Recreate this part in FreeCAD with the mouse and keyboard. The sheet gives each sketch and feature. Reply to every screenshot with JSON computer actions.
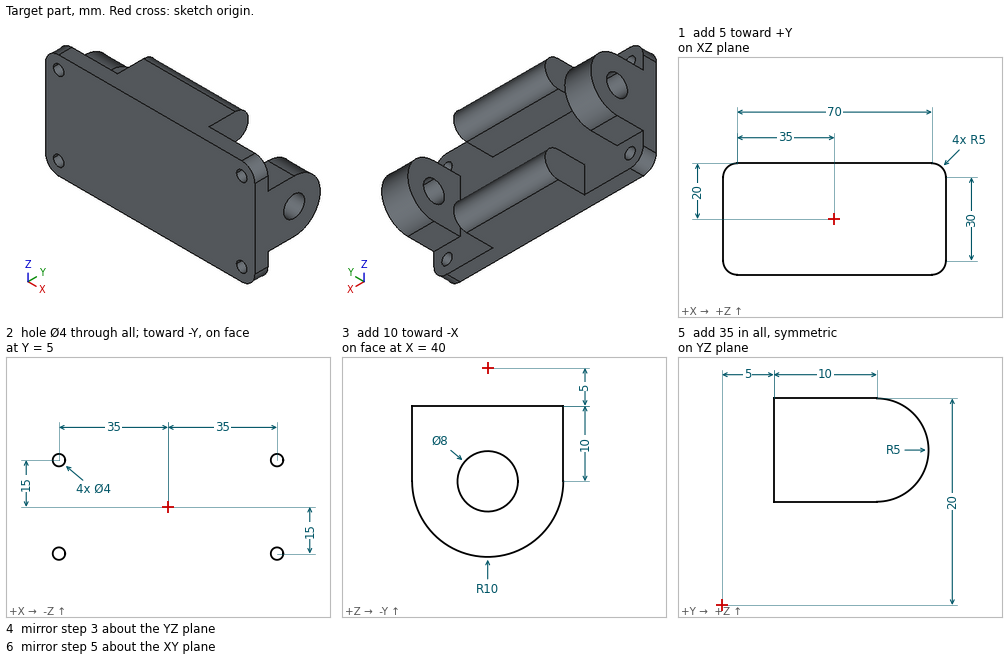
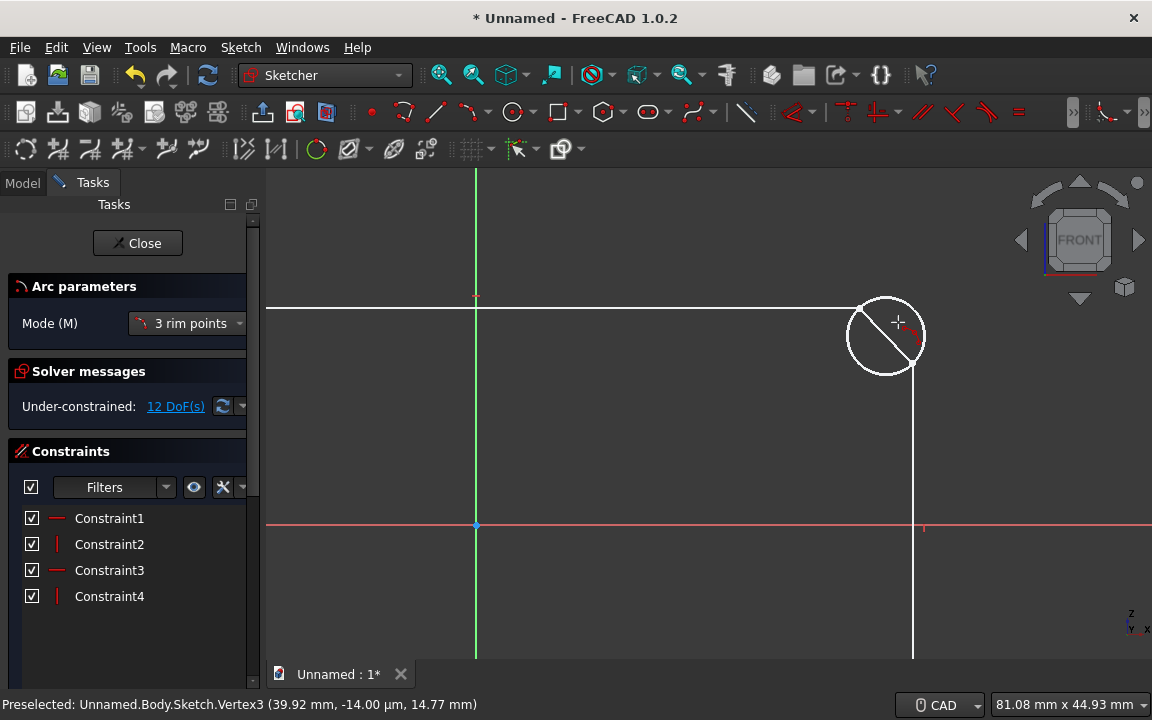
{"action": "left_click", "coordinate": [898, 323]}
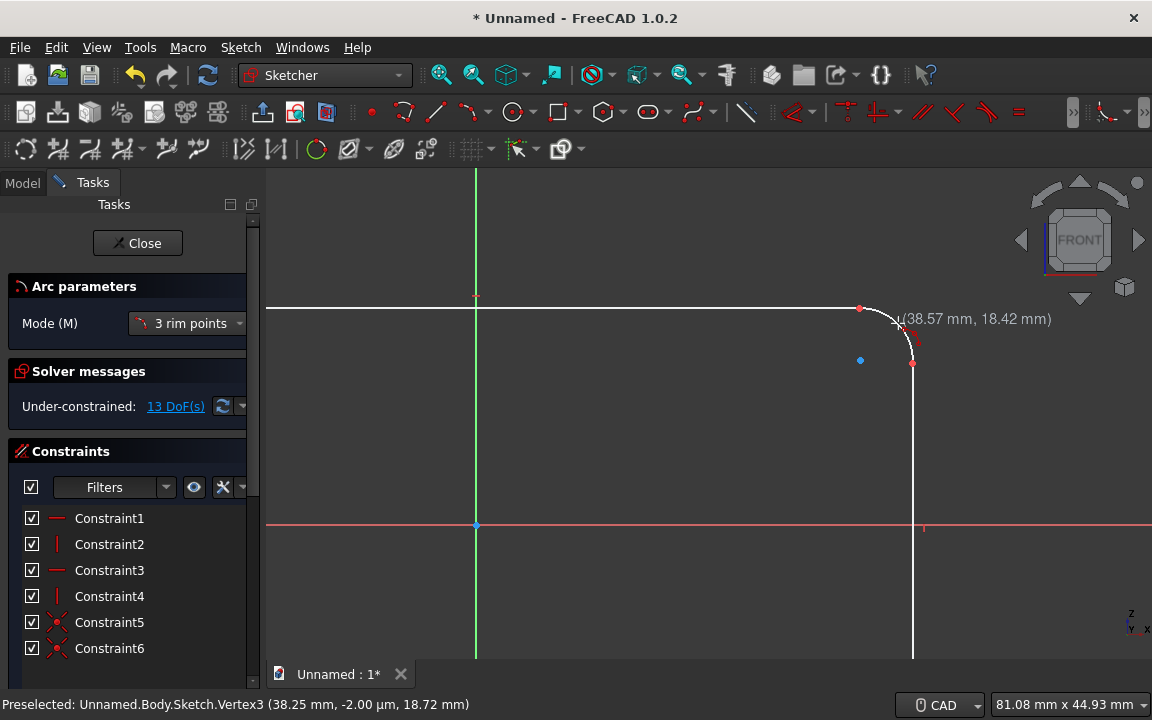
{"action": "scroll", "coordinate": [840, 278], "scroll_direction": "down", "scroll_amount": 3}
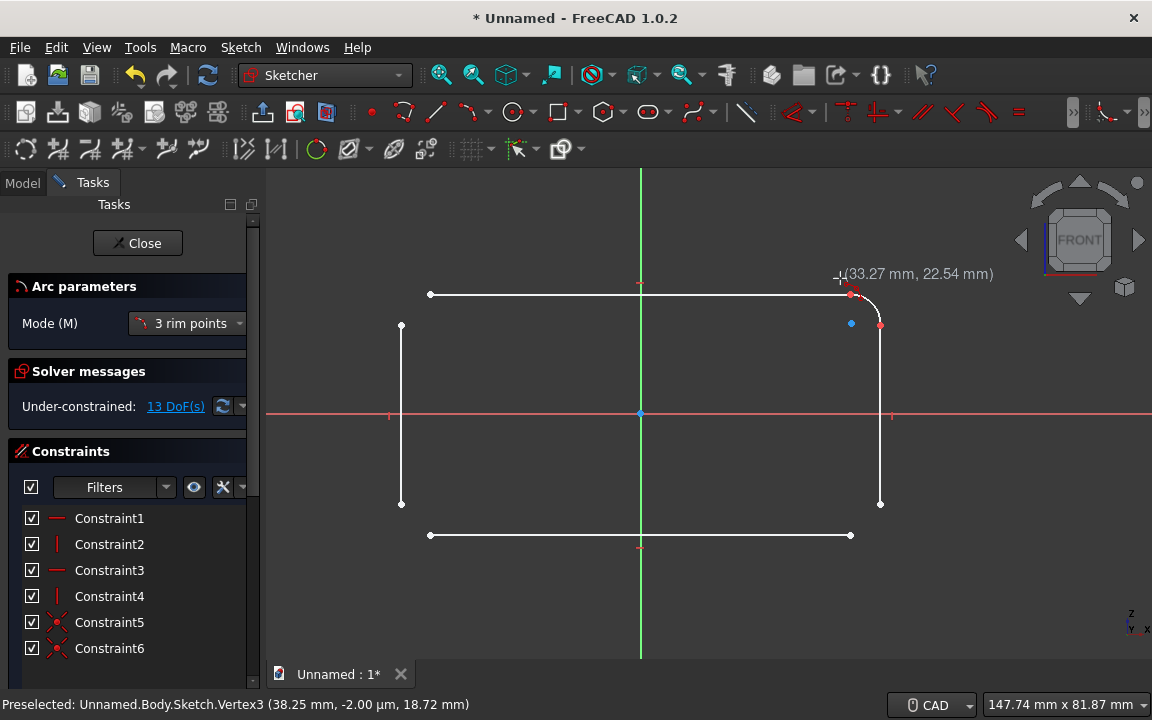
{"action": "left_click", "coordinate": [880, 505]}
{"action": "left_click", "coordinate": [851, 535]}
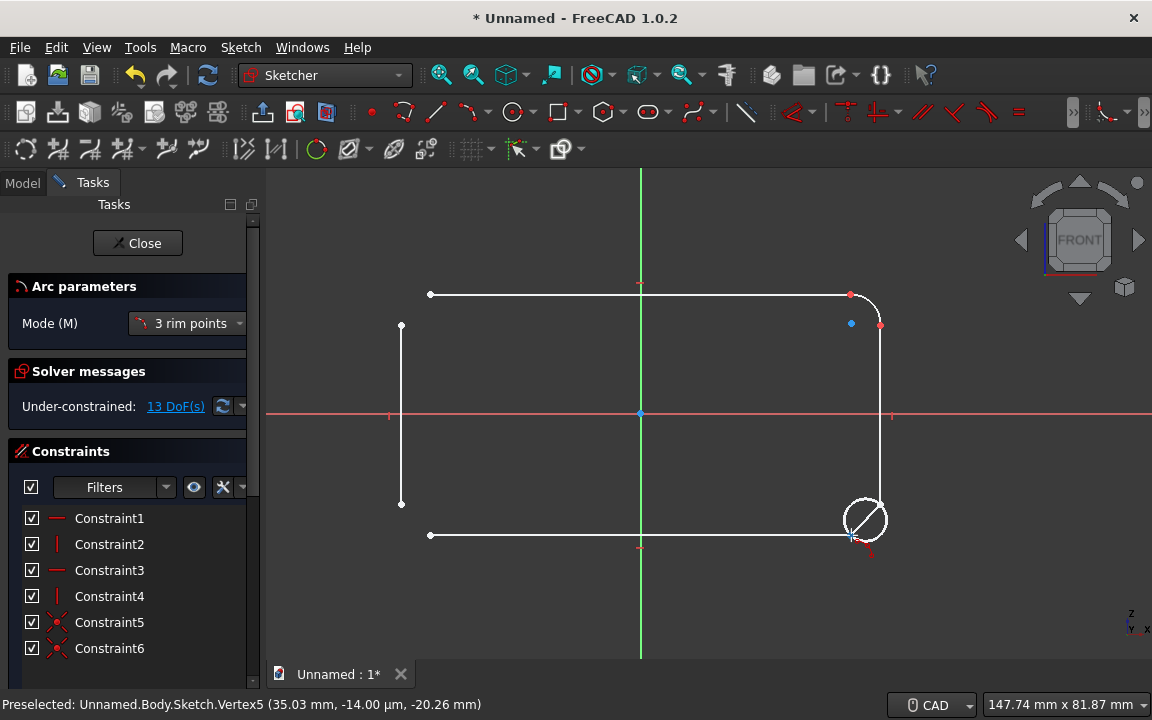
{"action": "scroll", "coordinate": [872, 525], "scroll_direction": "up", "scroll_amount": 3}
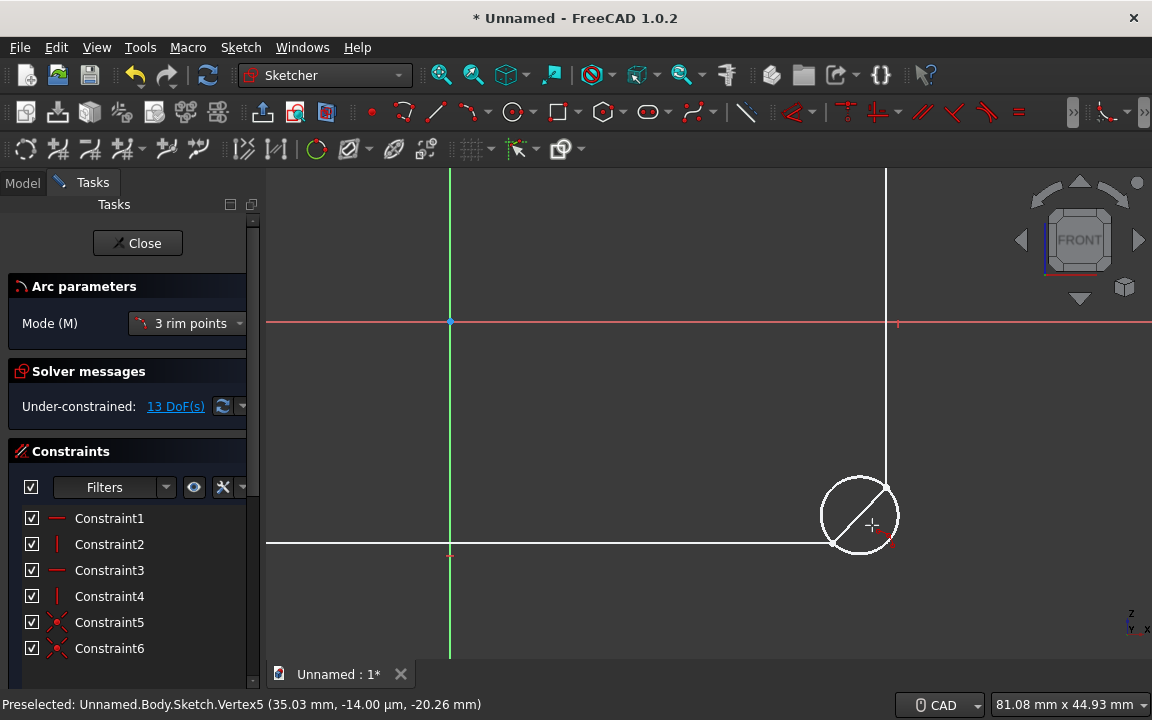
{"action": "left_click", "coordinate": [871, 524]}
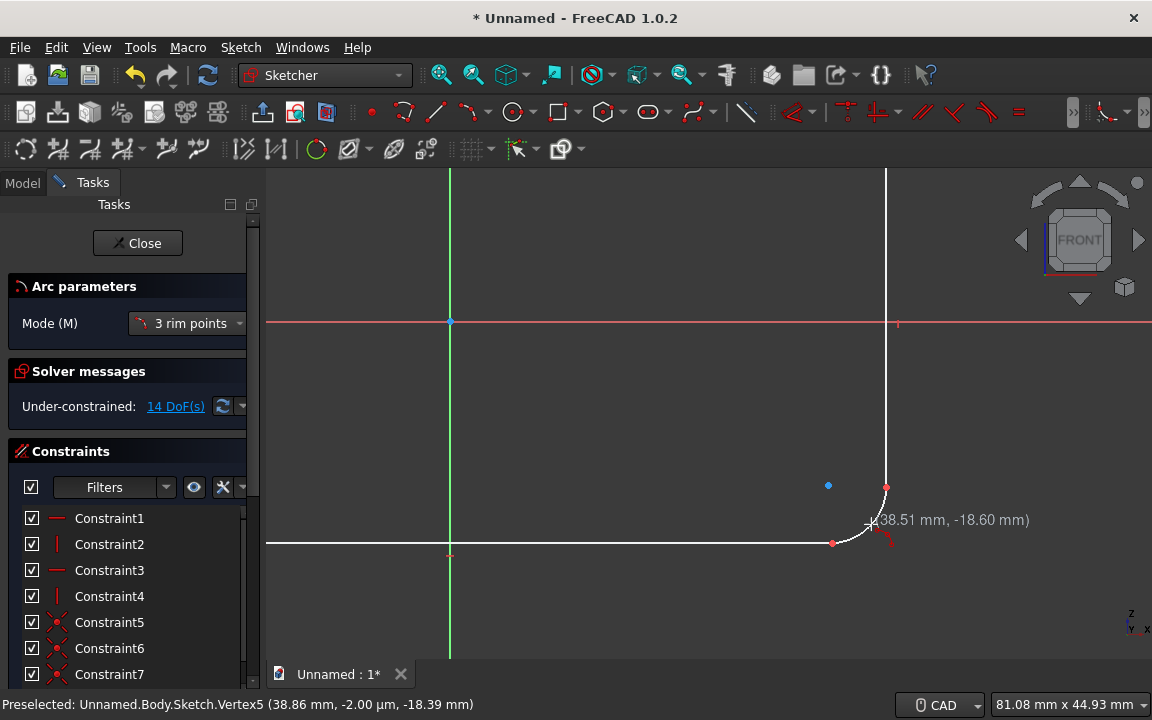
{"action": "scroll", "coordinate": [872, 525], "scroll_direction": "down", "scroll_amount": 3}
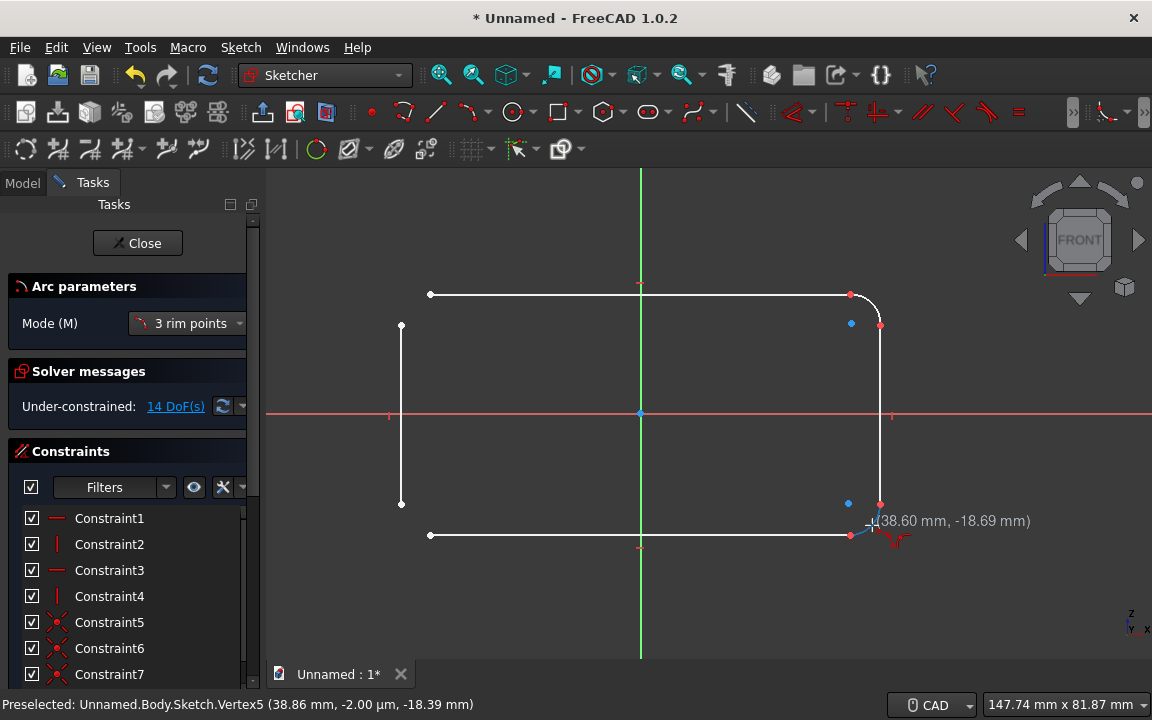
{"action": "left_click", "coordinate": [431, 535]}
{"action": "left_click", "coordinate": [401, 505]}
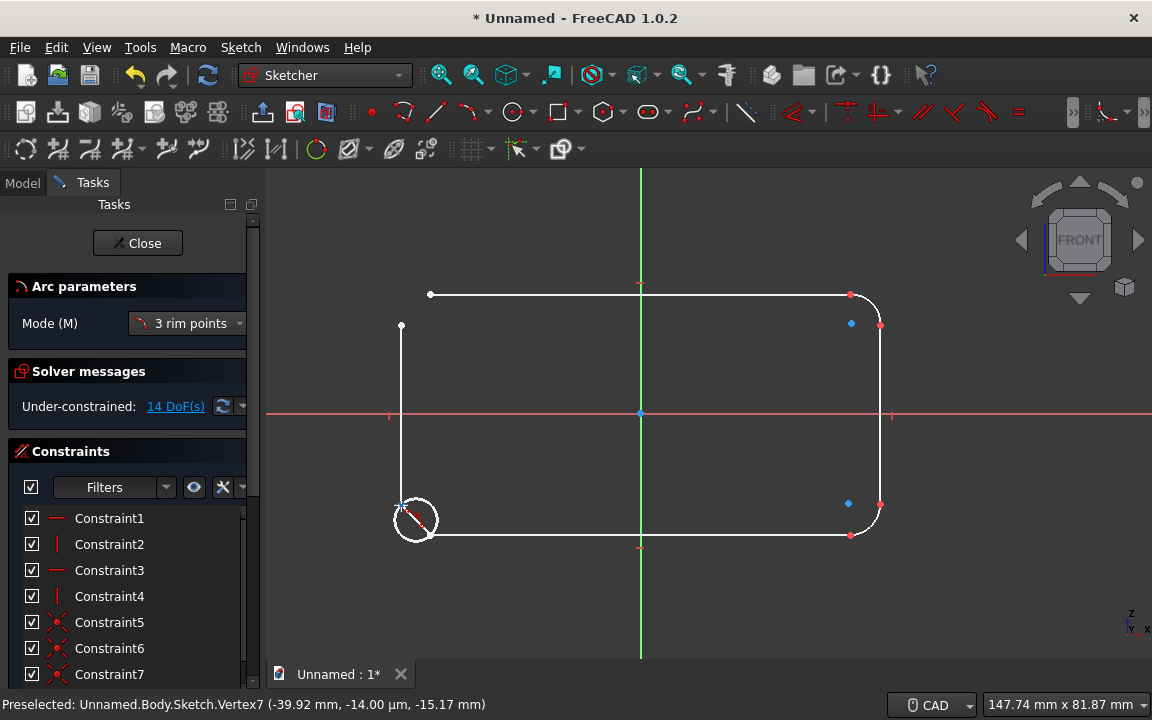
{"action": "scroll", "coordinate": [410, 525], "scroll_direction": "up", "scroll_amount": 3}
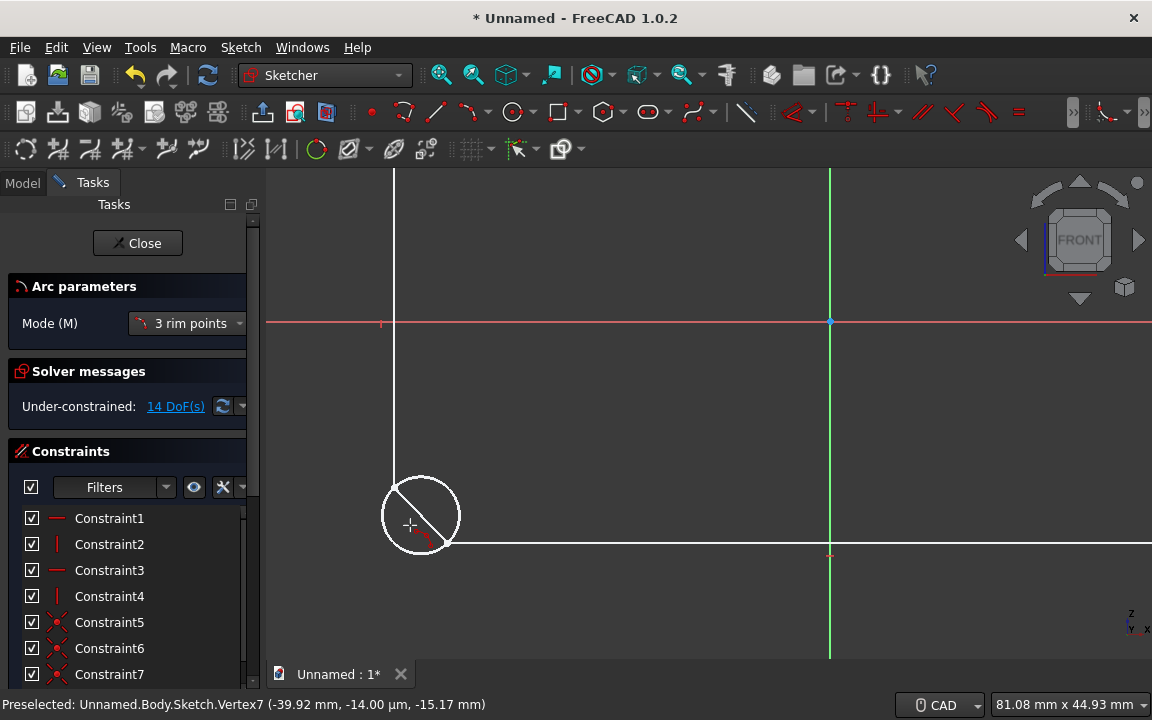
{"action": "left_click", "coordinate": [409, 524]}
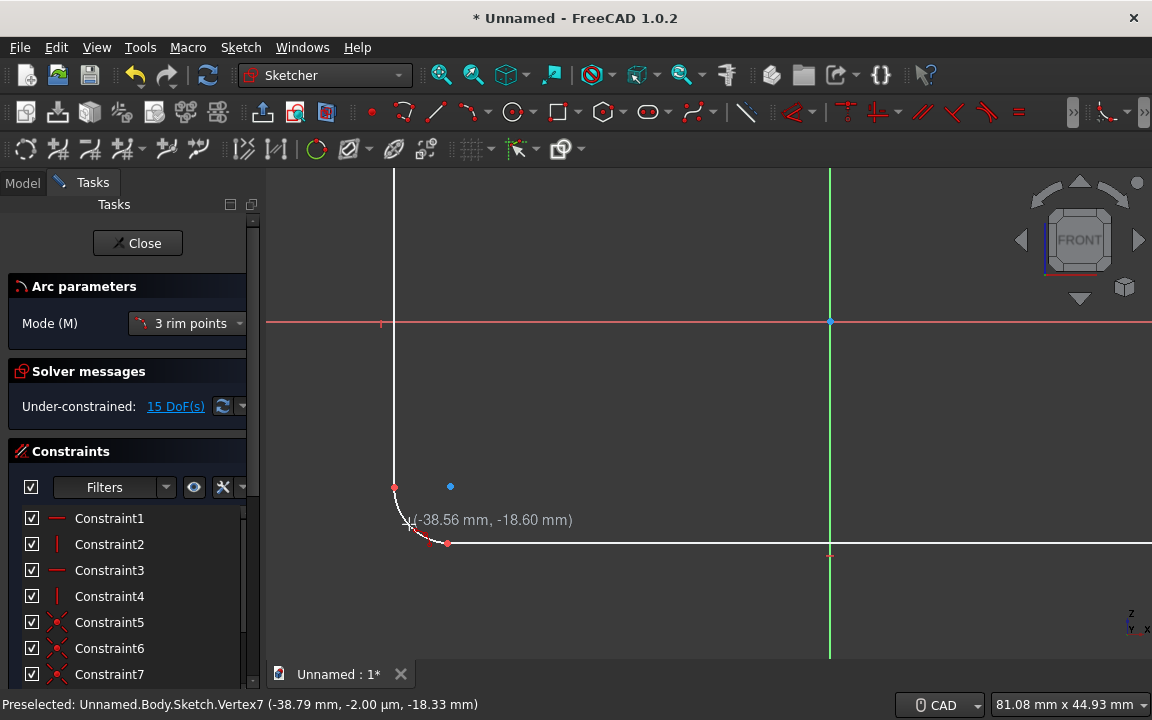
{"action": "scroll", "coordinate": [410, 525], "scroll_direction": "down", "scroll_amount": 3}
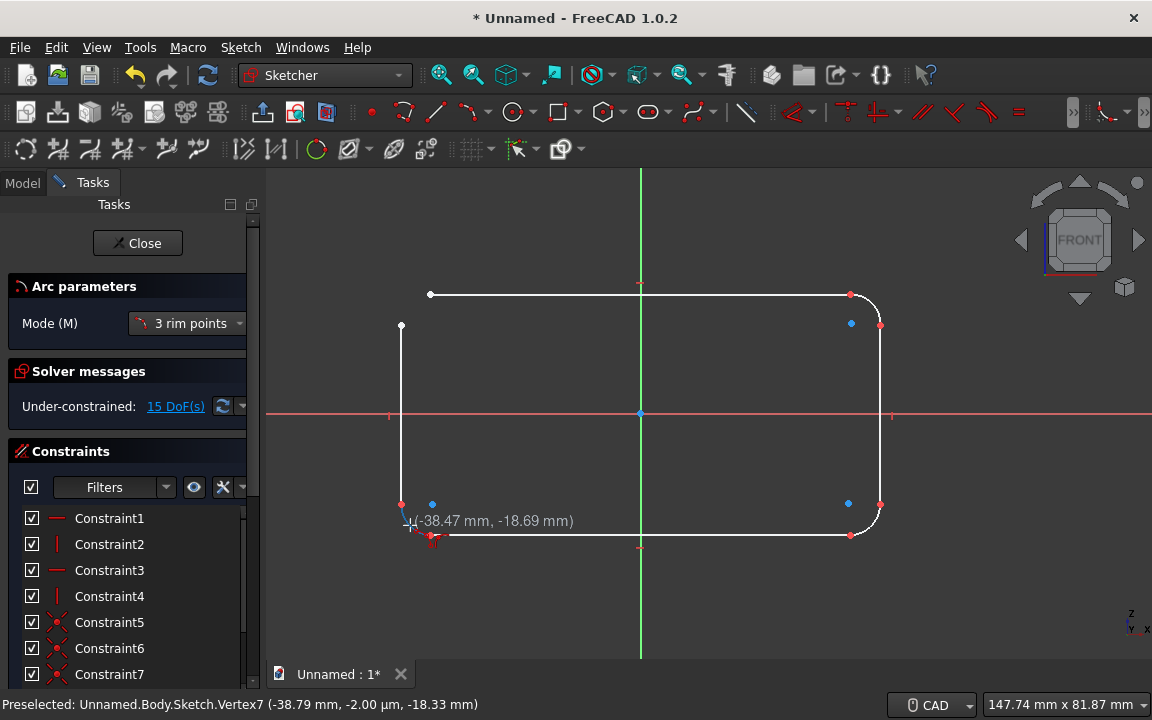
{"action": "left_click", "coordinate": [401, 325]}
{"action": "left_click", "coordinate": [431, 295]}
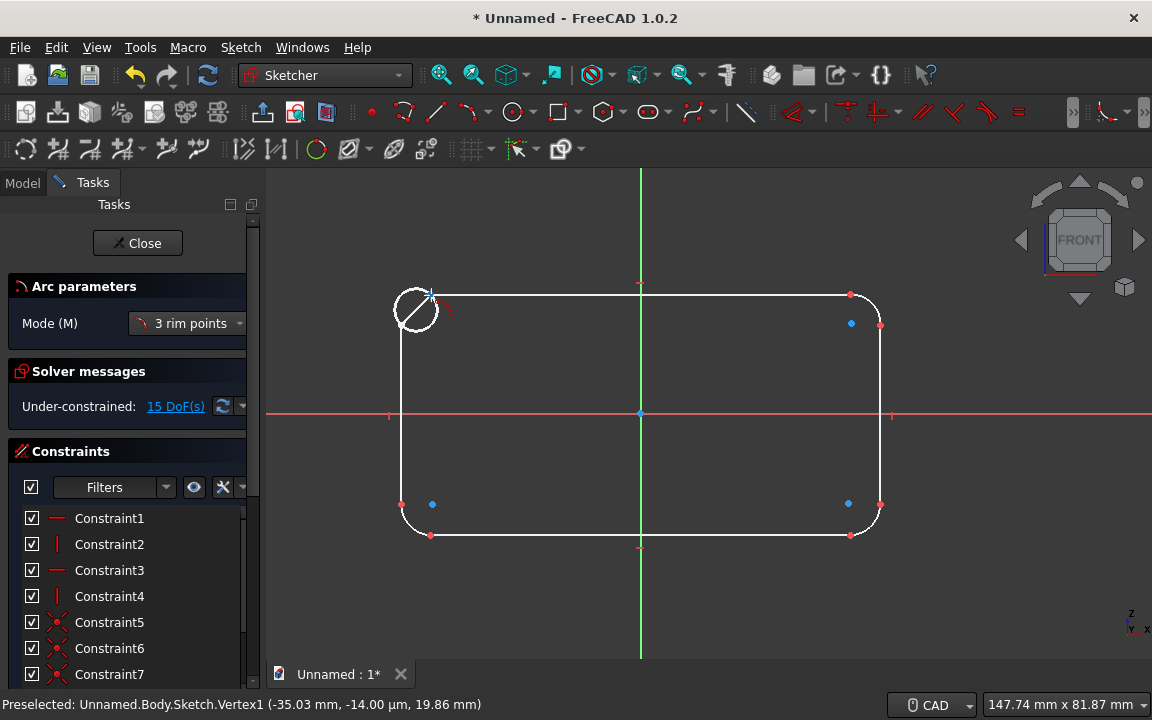
{"action": "scroll", "coordinate": [410, 303], "scroll_direction": "up", "scroll_amount": 3}